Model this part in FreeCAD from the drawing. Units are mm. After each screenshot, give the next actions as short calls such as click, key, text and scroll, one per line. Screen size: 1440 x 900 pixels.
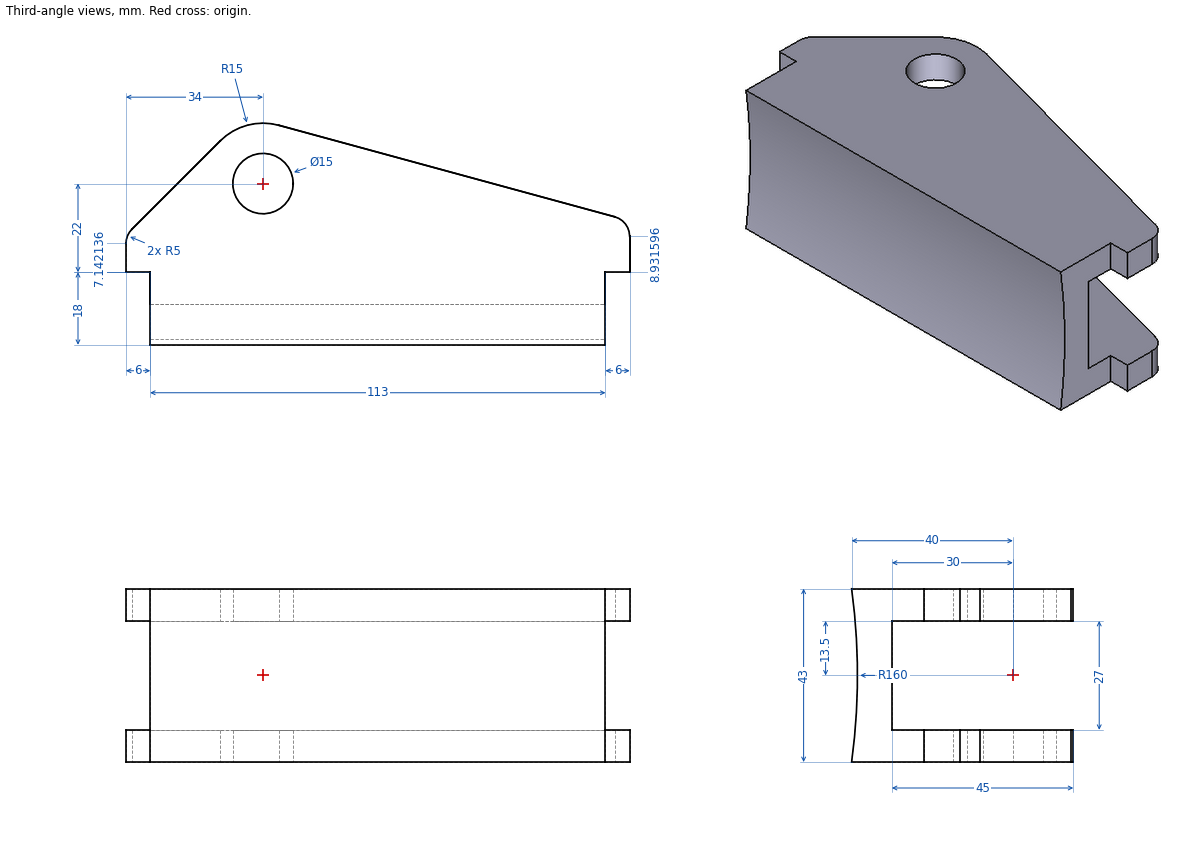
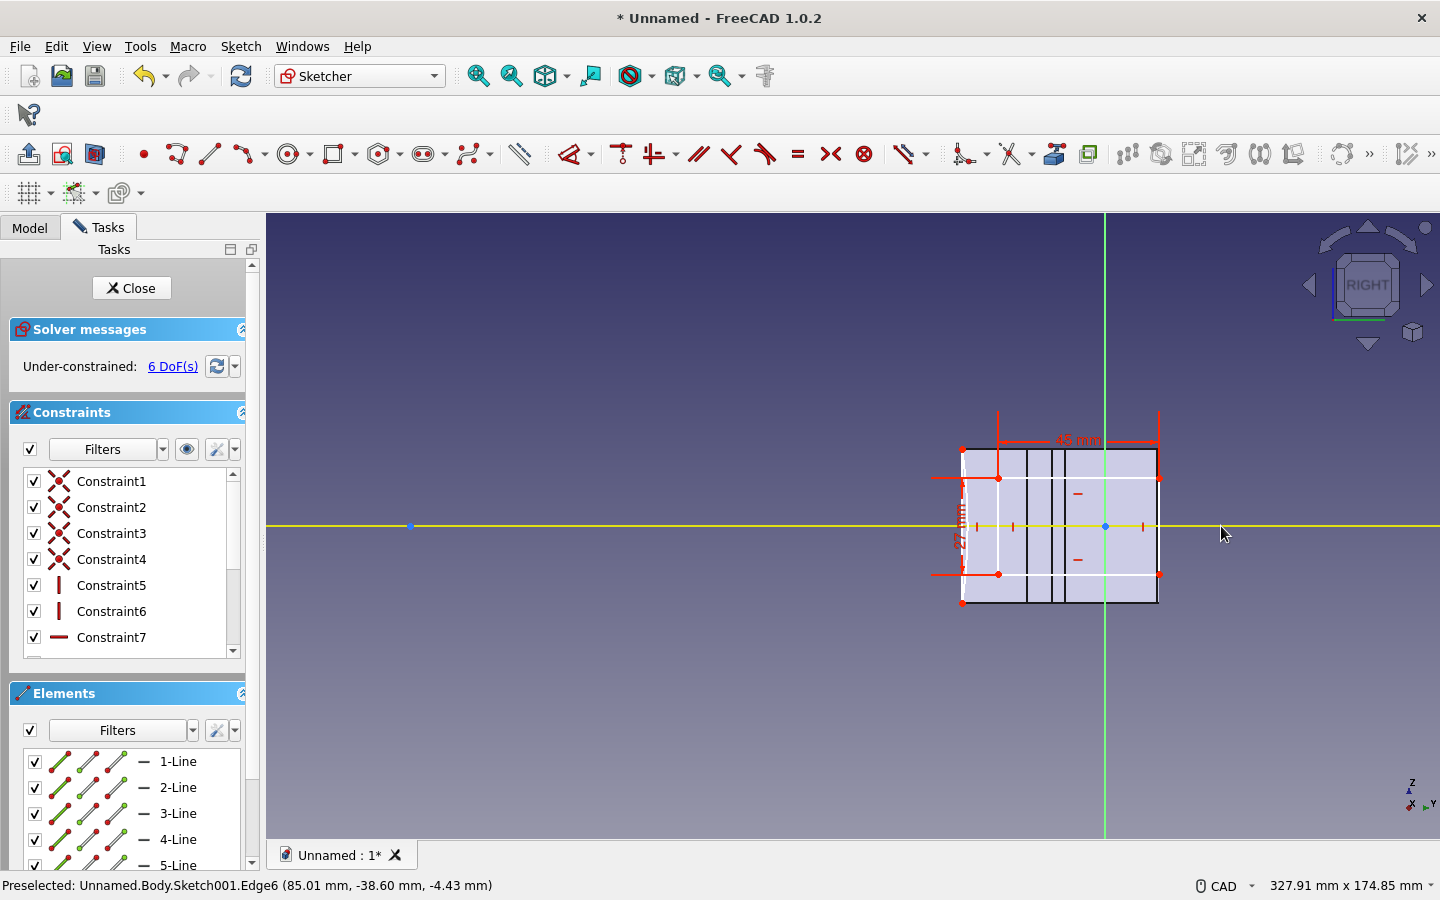
click(411, 527)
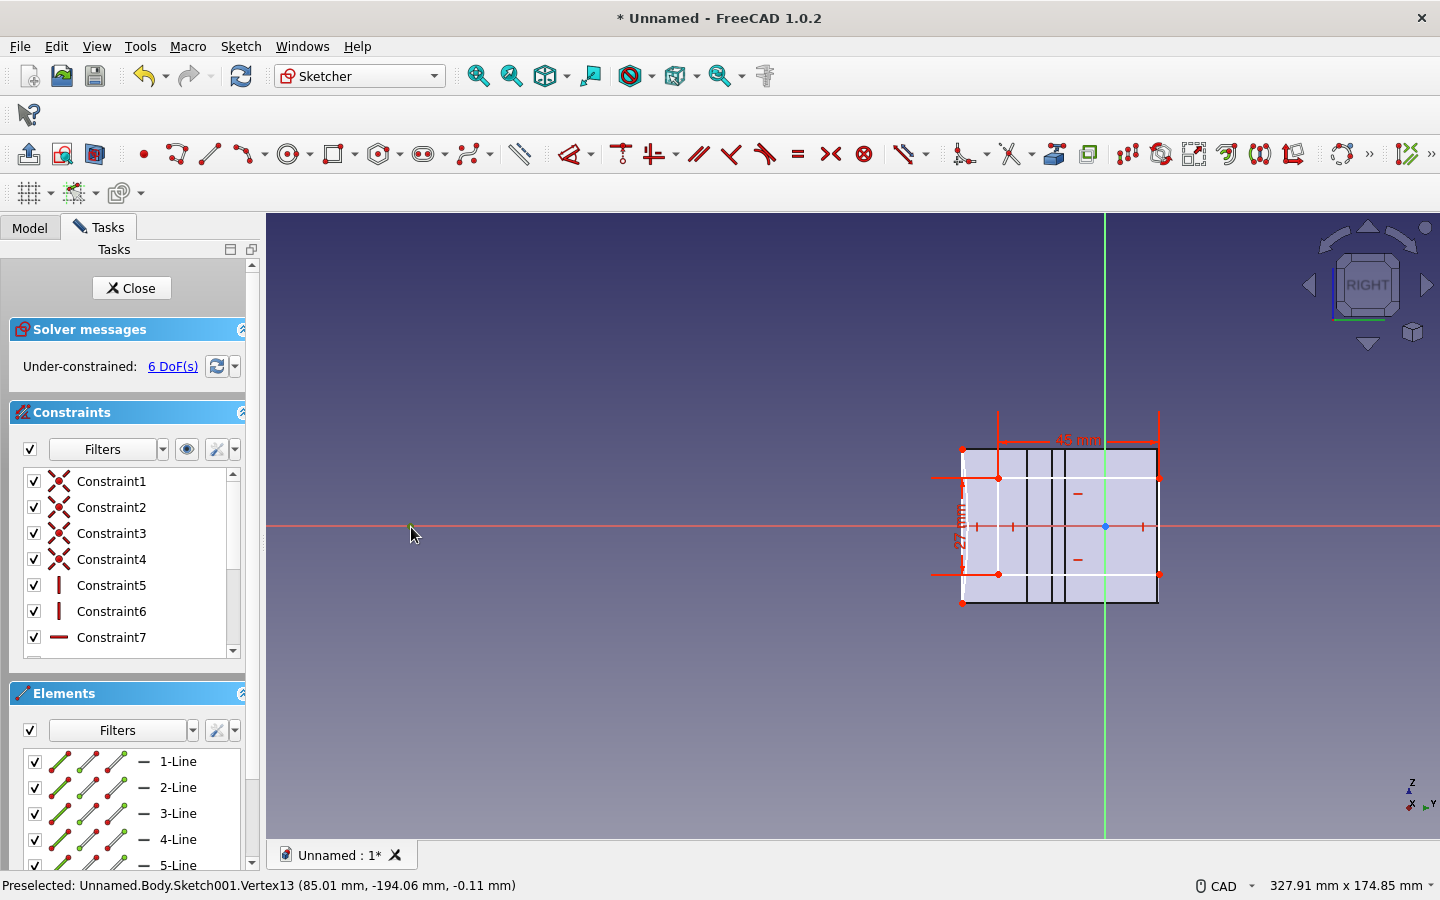
click(364, 526)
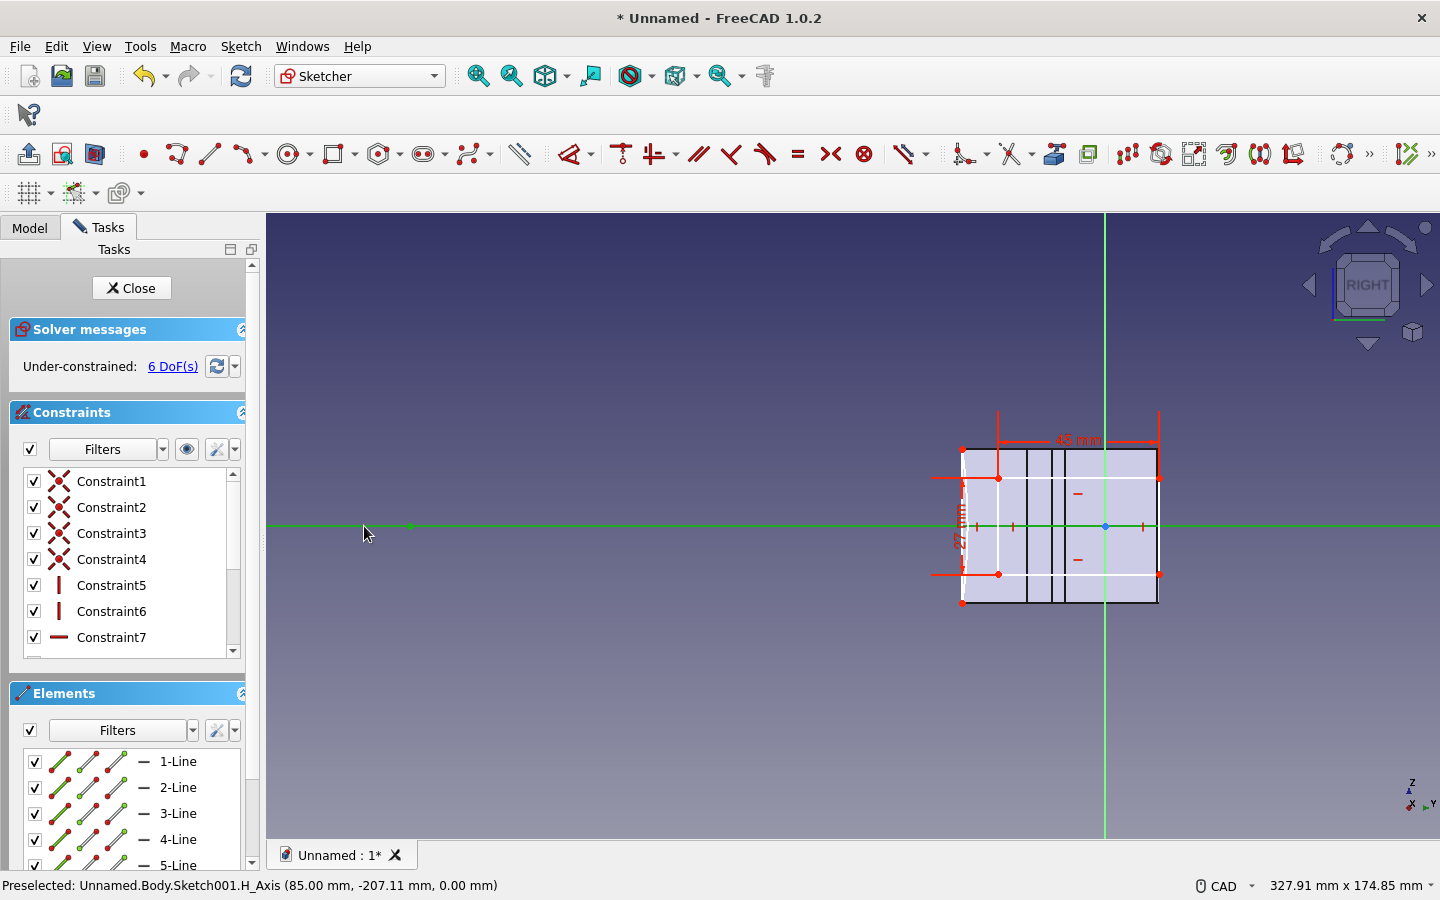
click(621, 154)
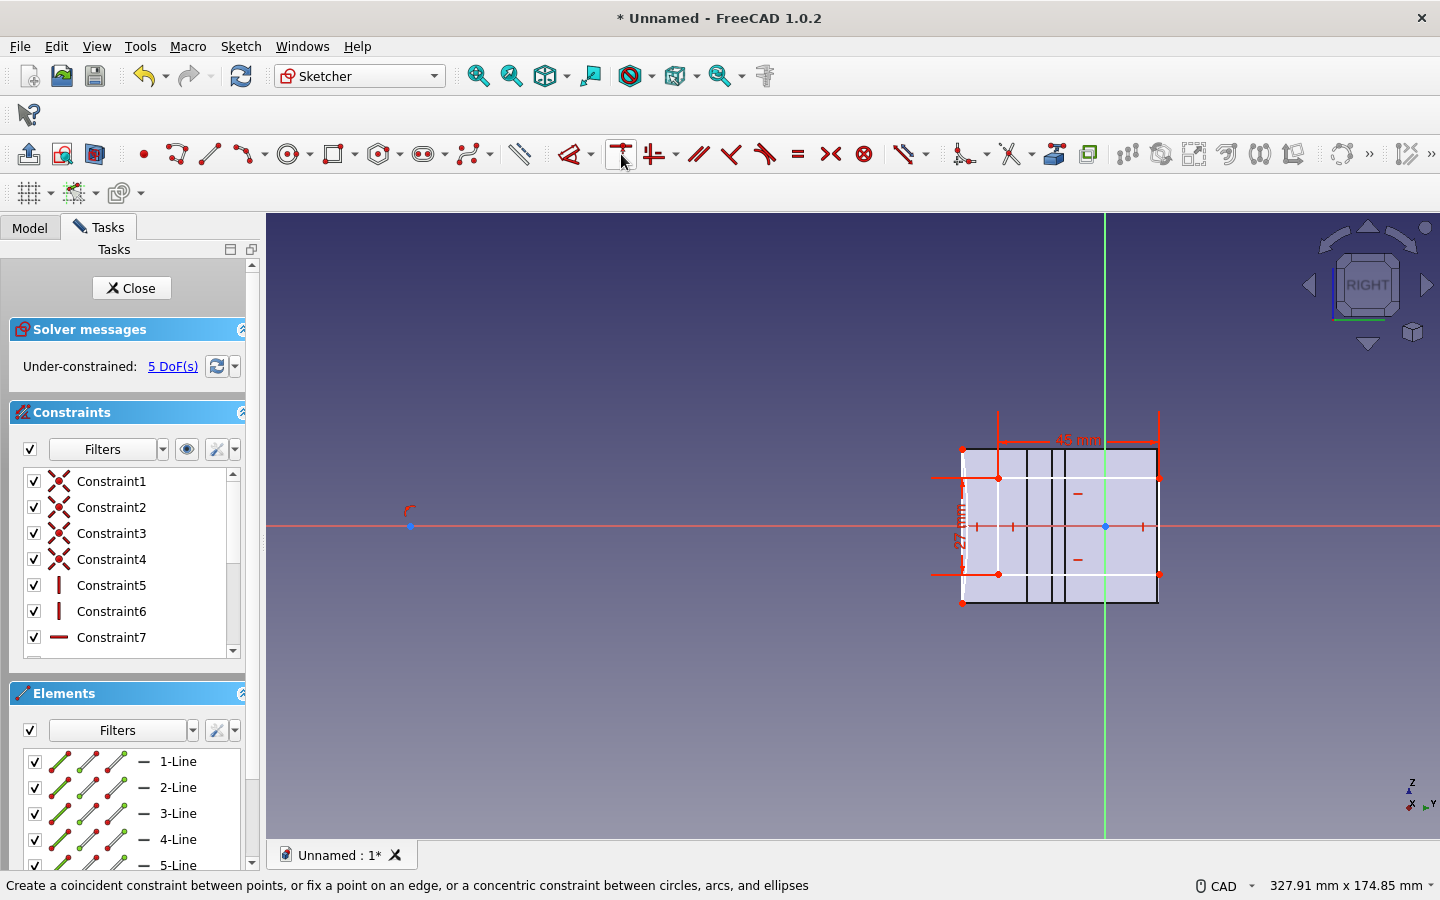
click(568, 154)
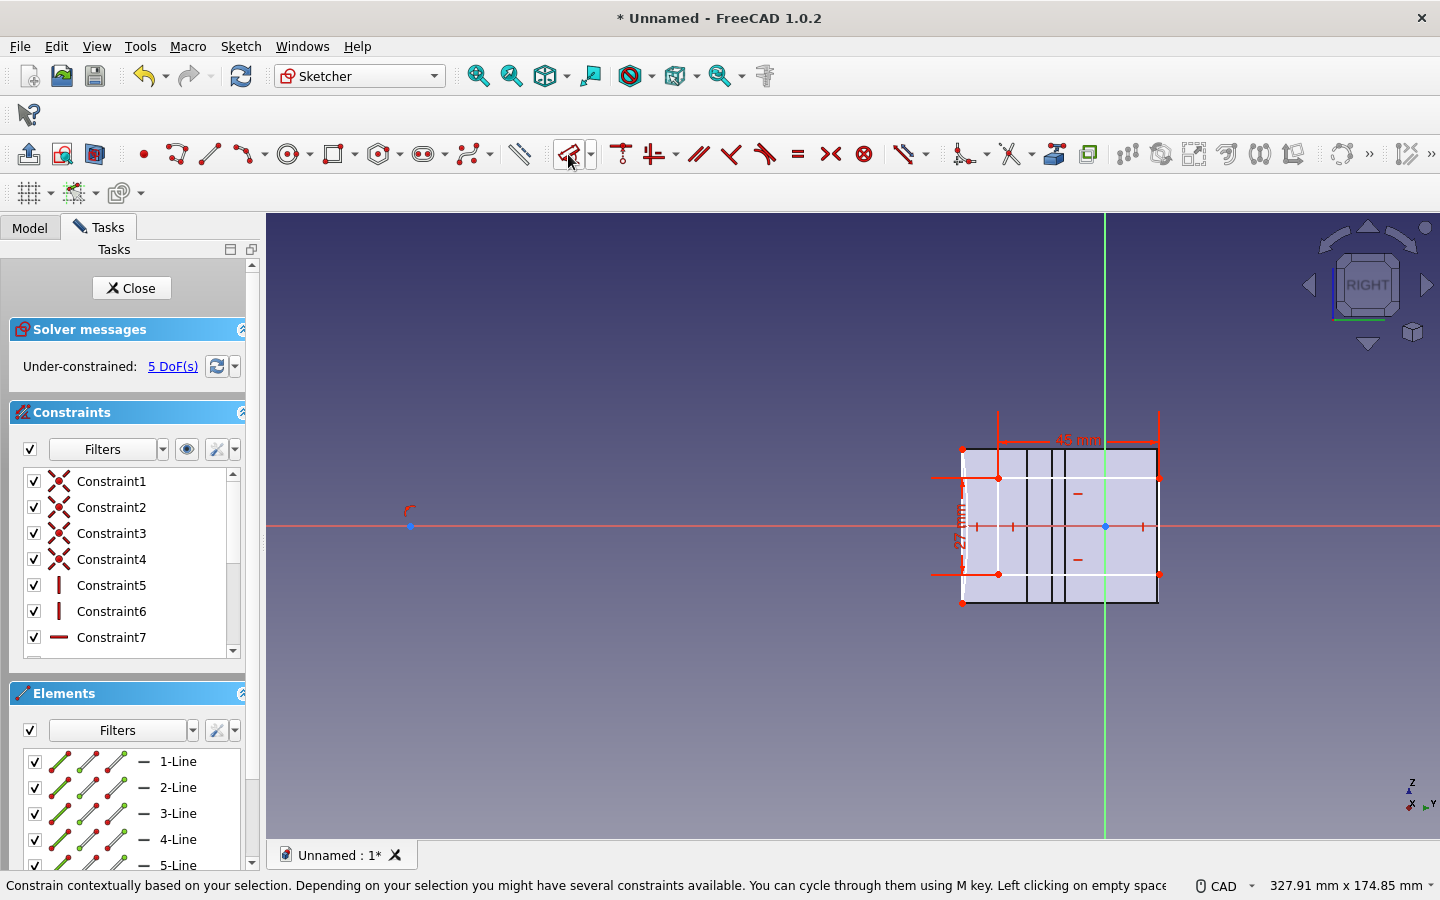
scroll(968, 526, up, 5)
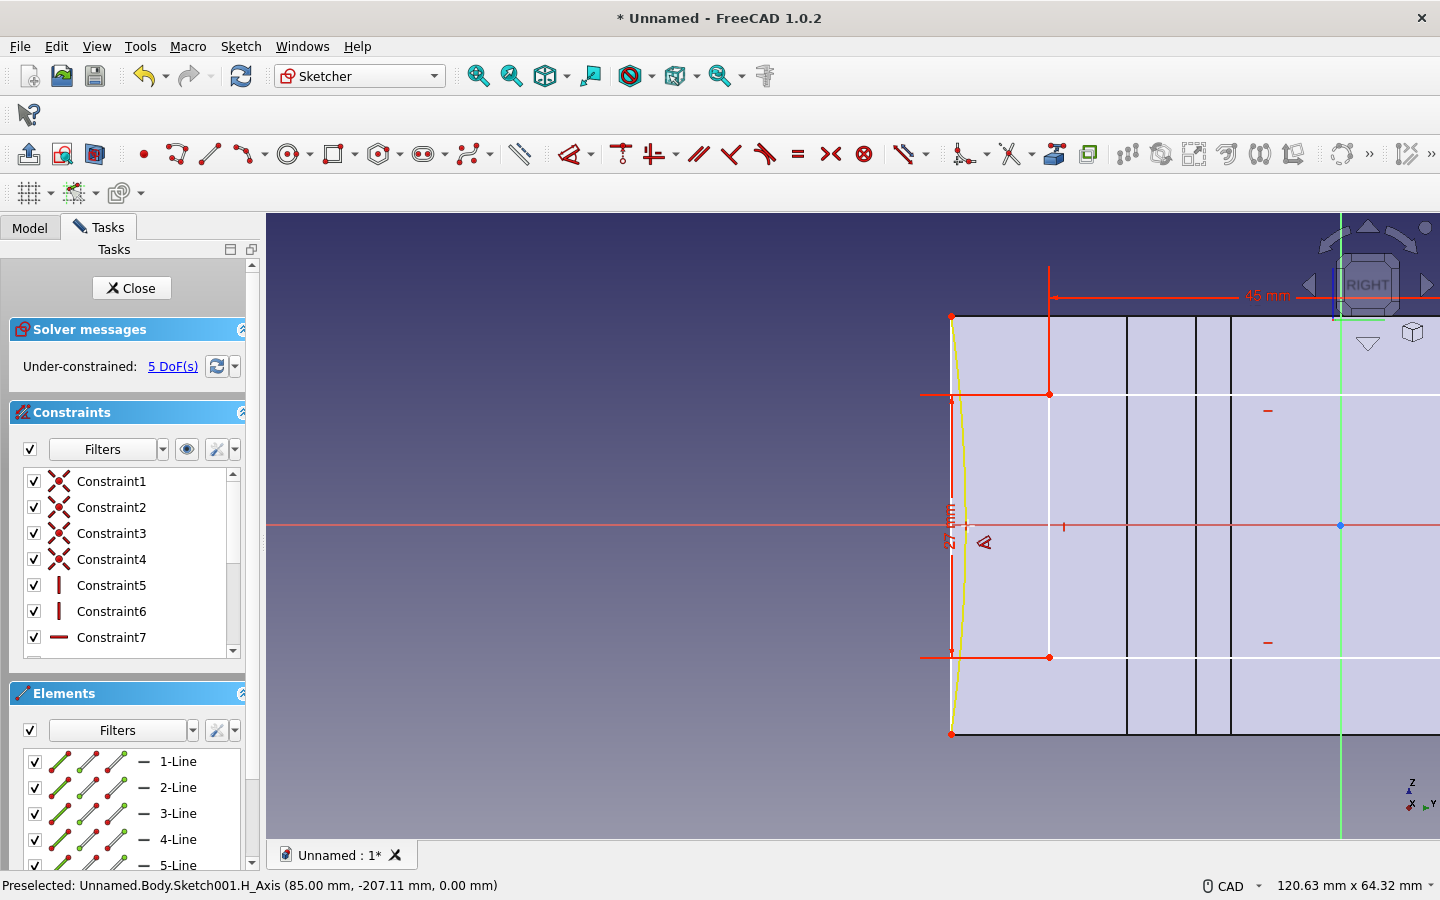
click(966, 525)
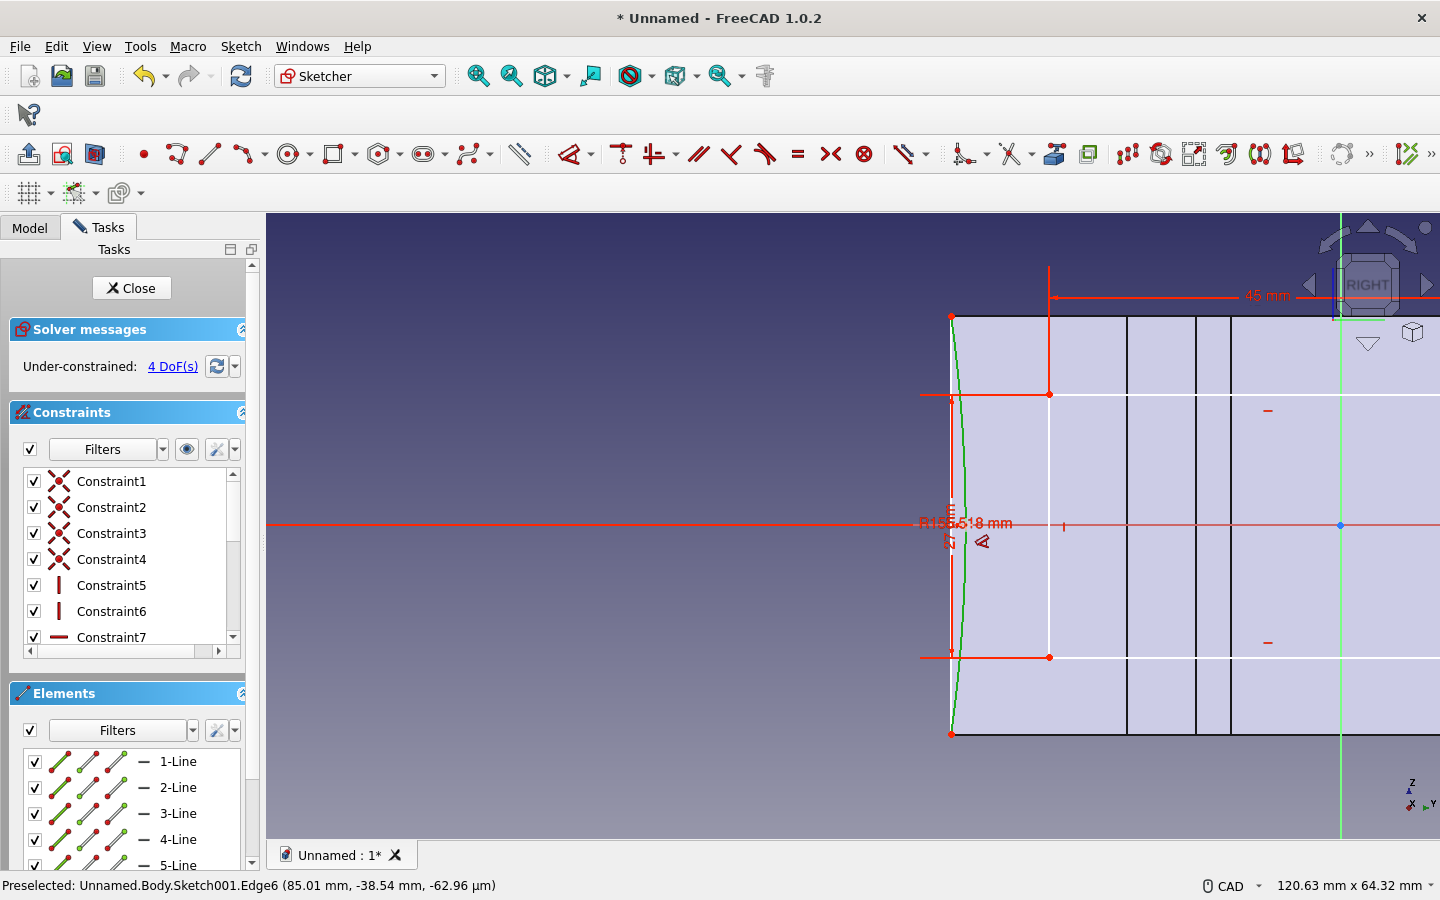
key(Escape)
key(Escape)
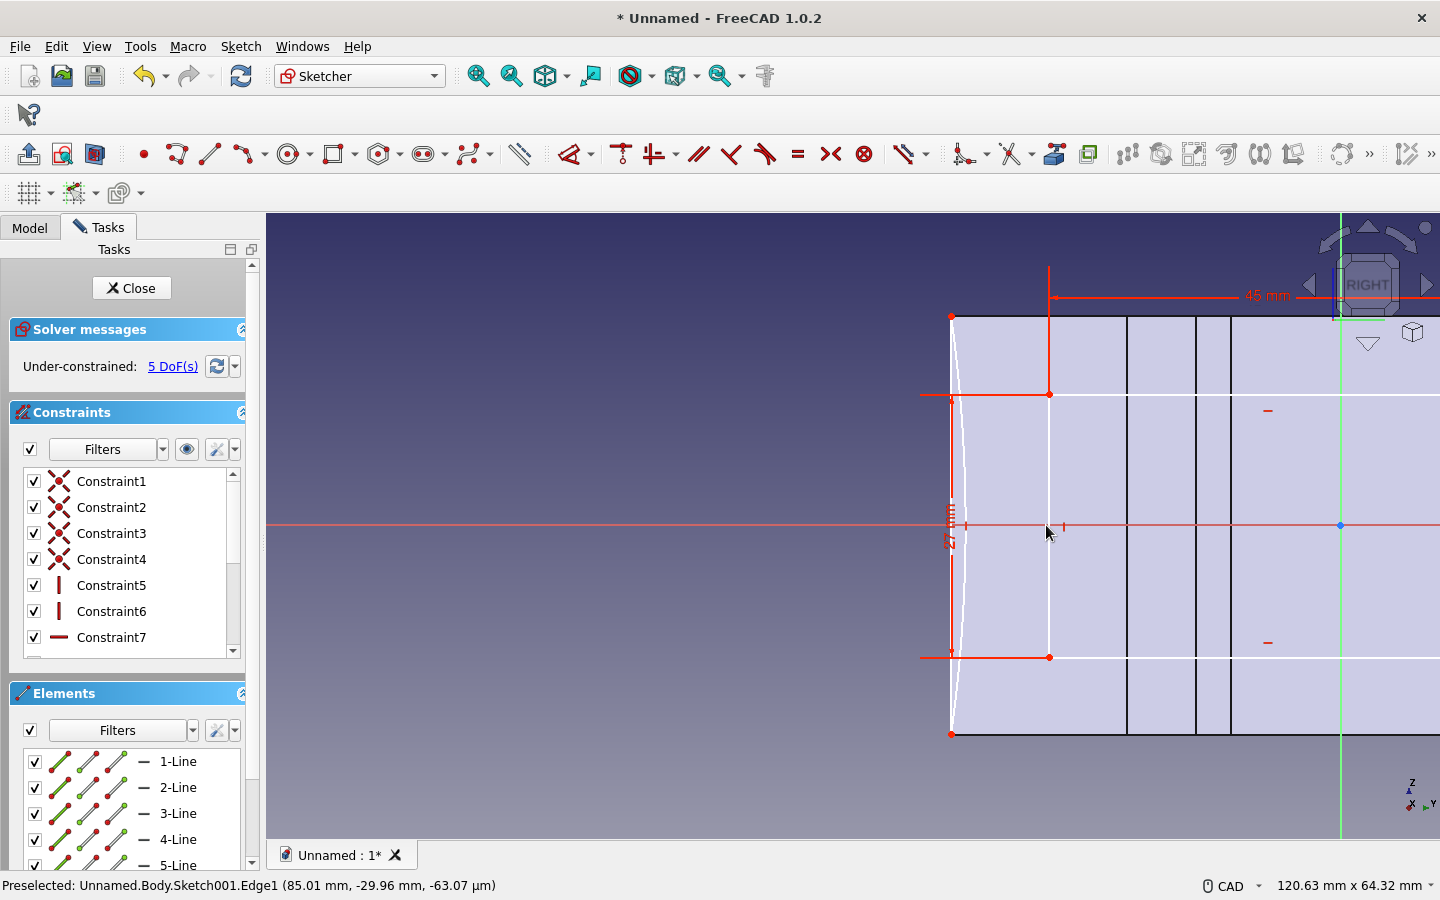
click(963, 609)